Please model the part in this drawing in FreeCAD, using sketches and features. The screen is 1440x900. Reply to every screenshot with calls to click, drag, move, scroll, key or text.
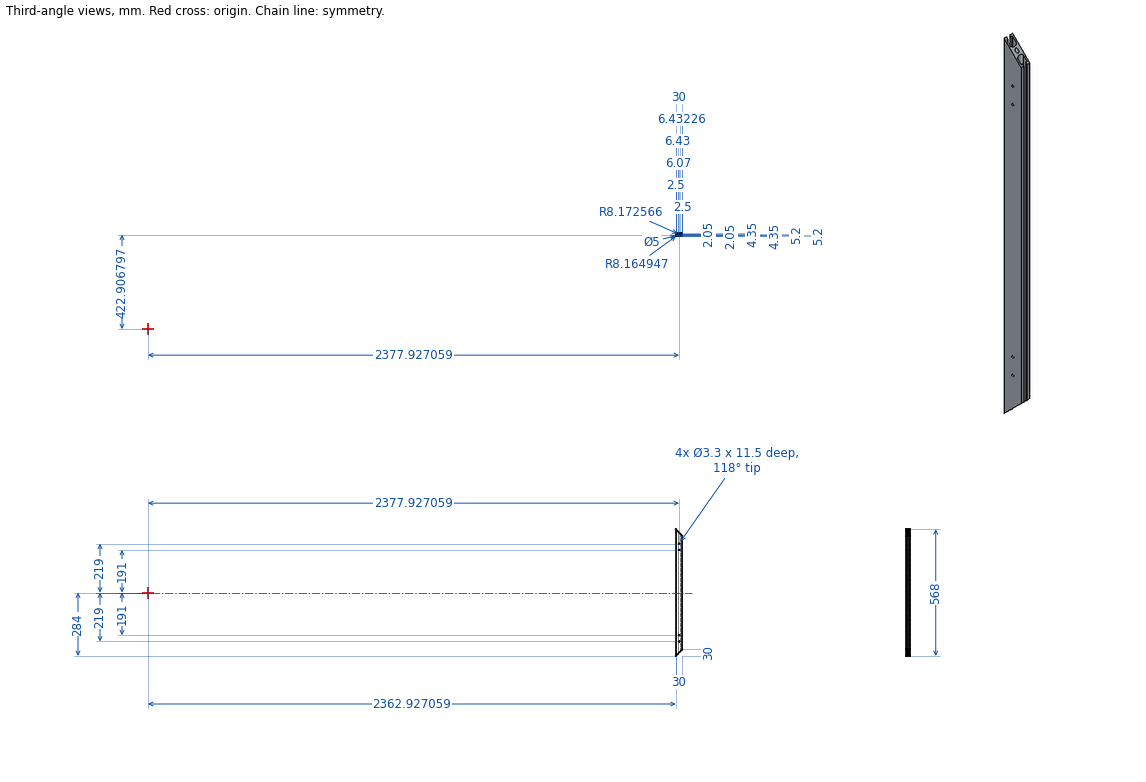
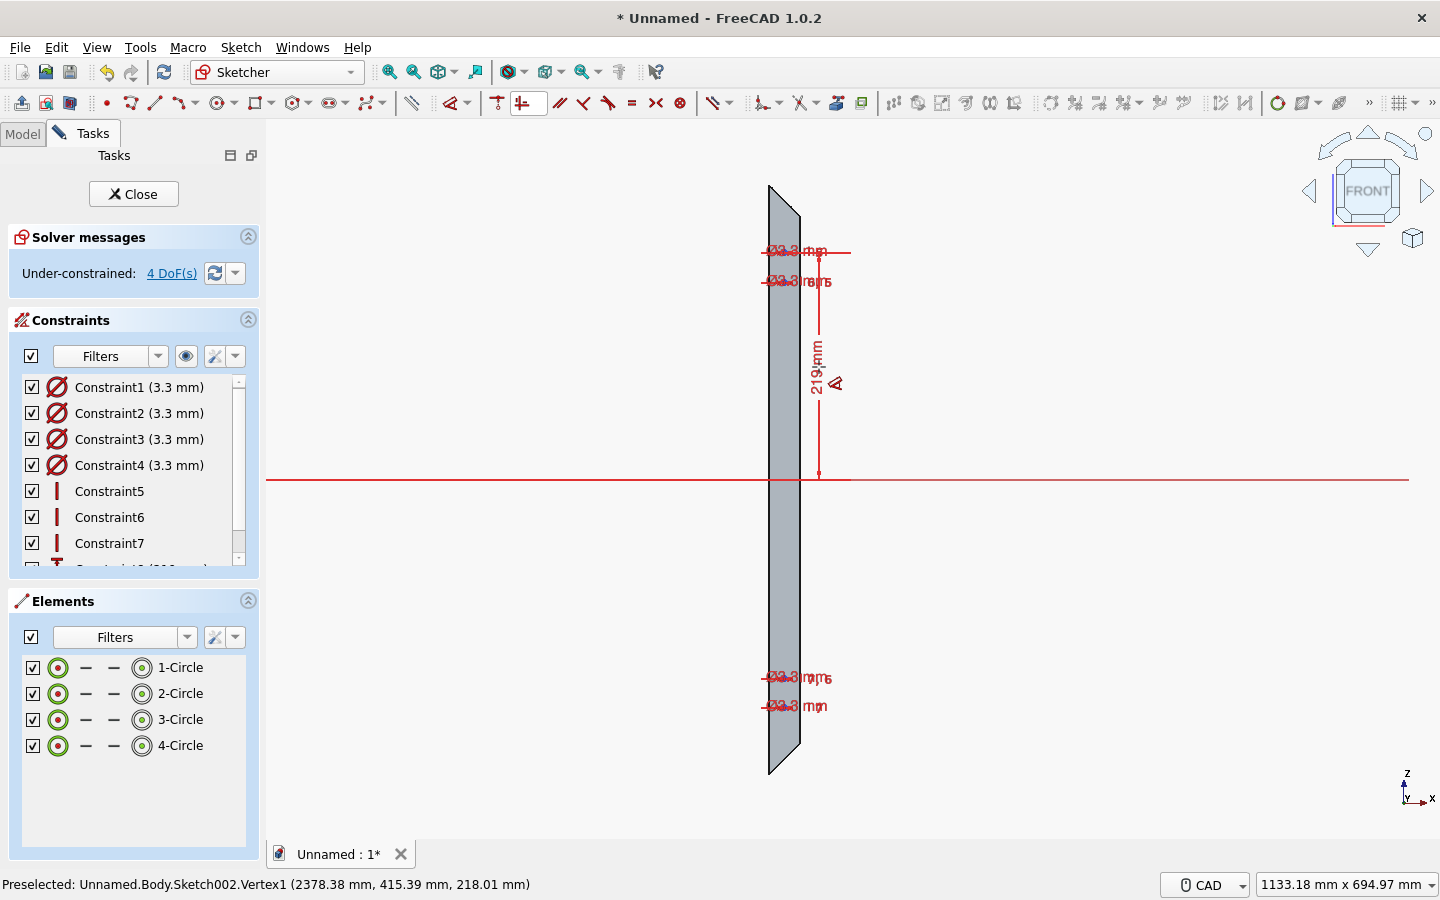
click(785, 283)
click(819, 336)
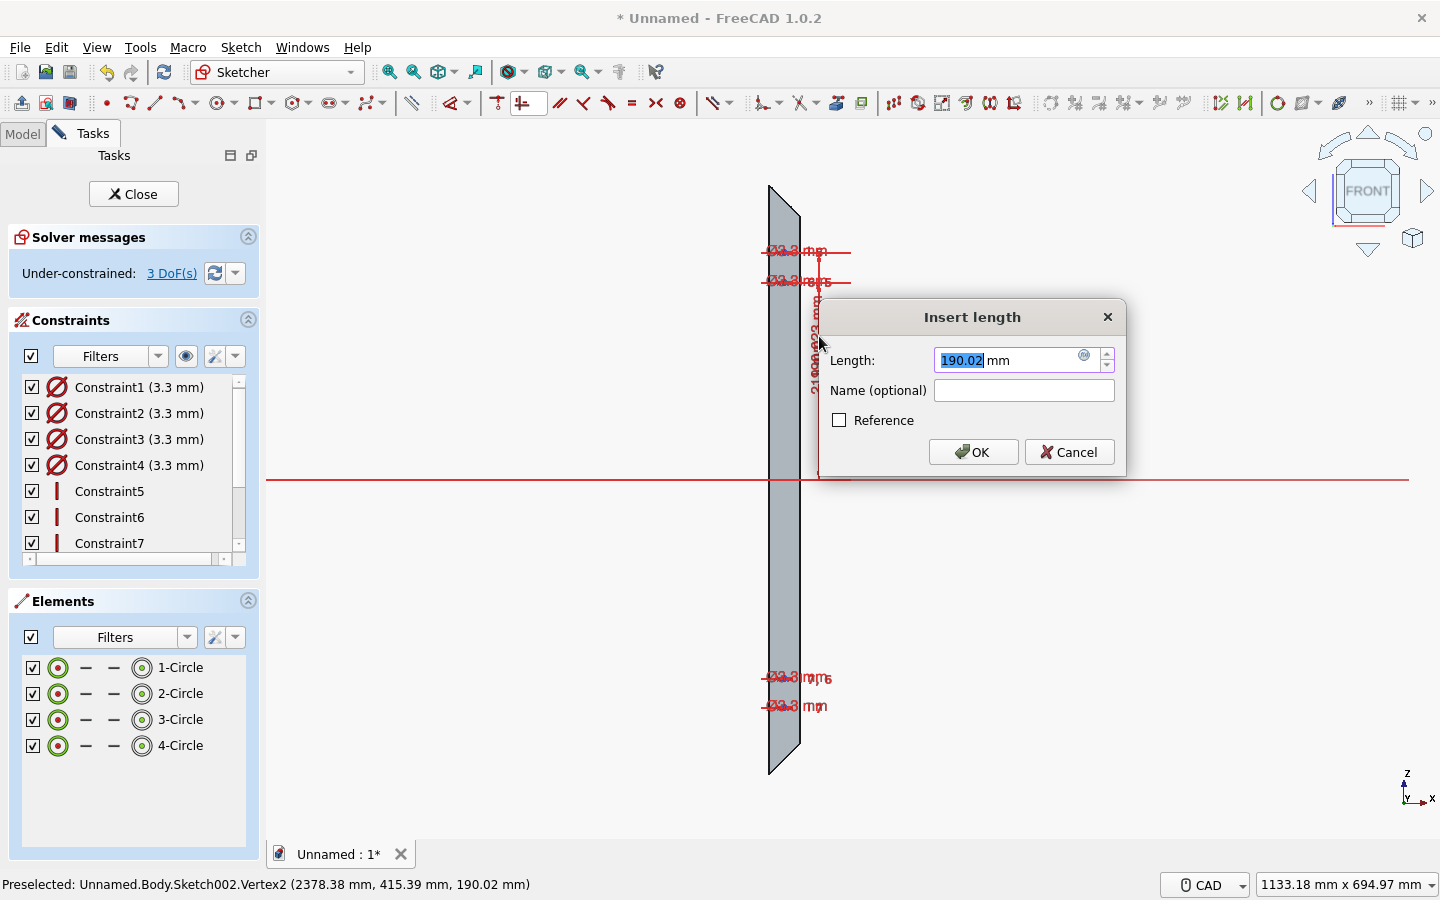
text(191)
key(Return)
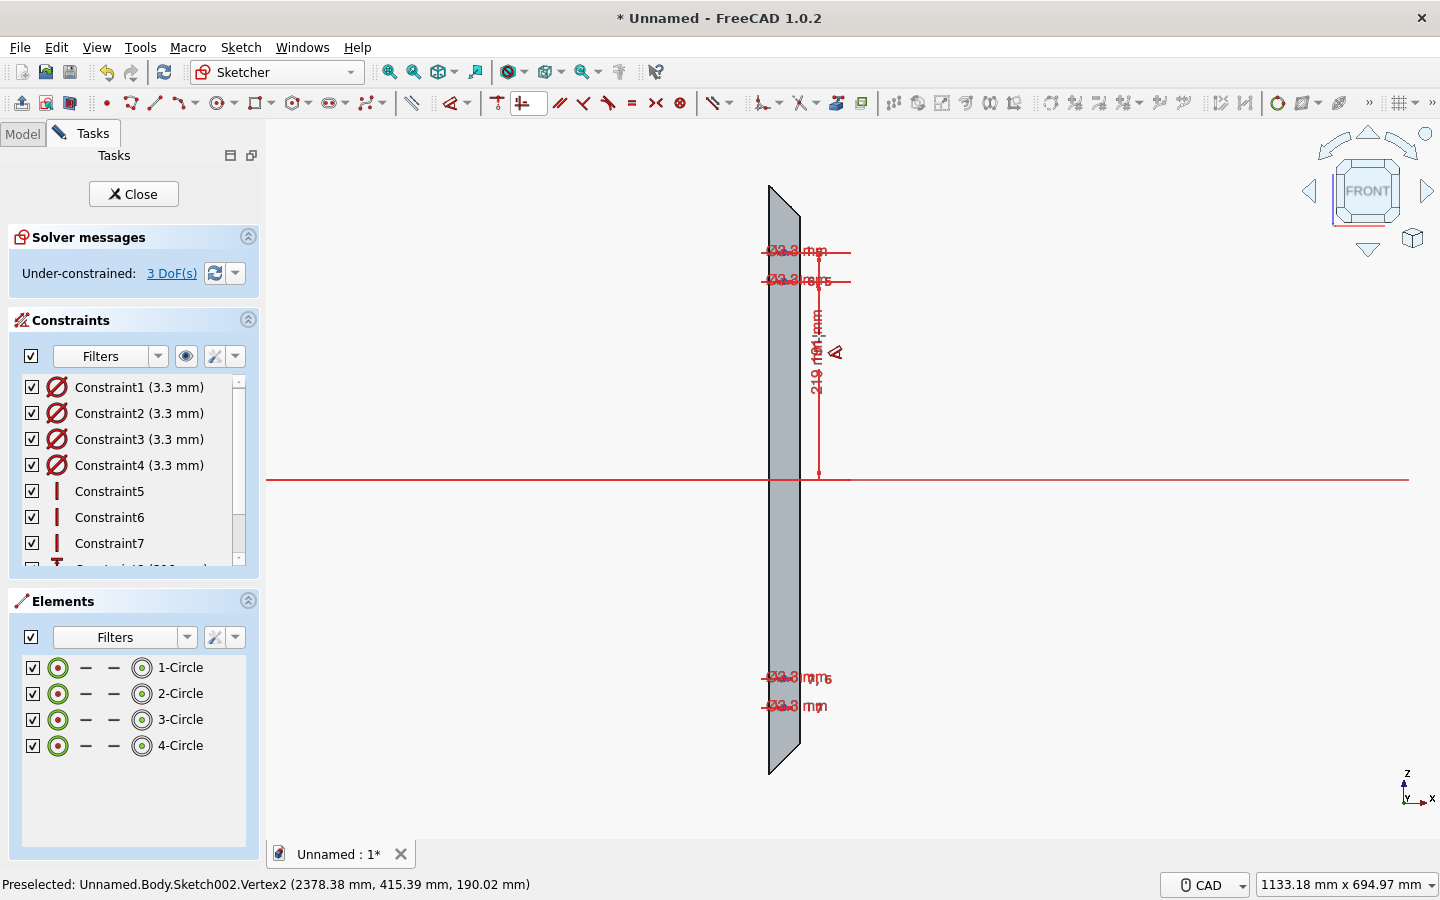
click(785, 679)
click(819, 579)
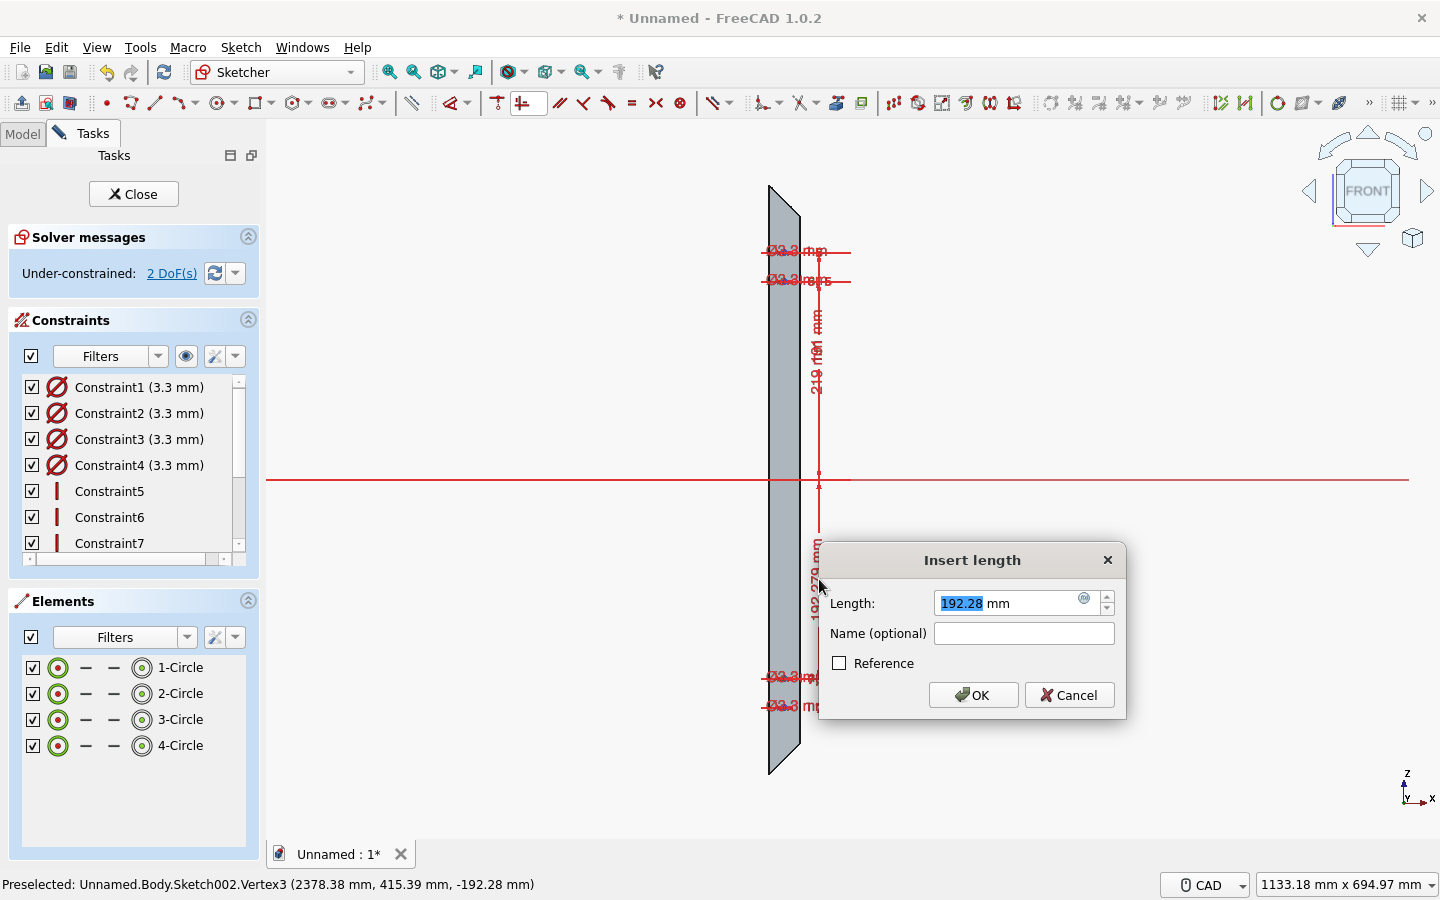
text(191)
key(Return)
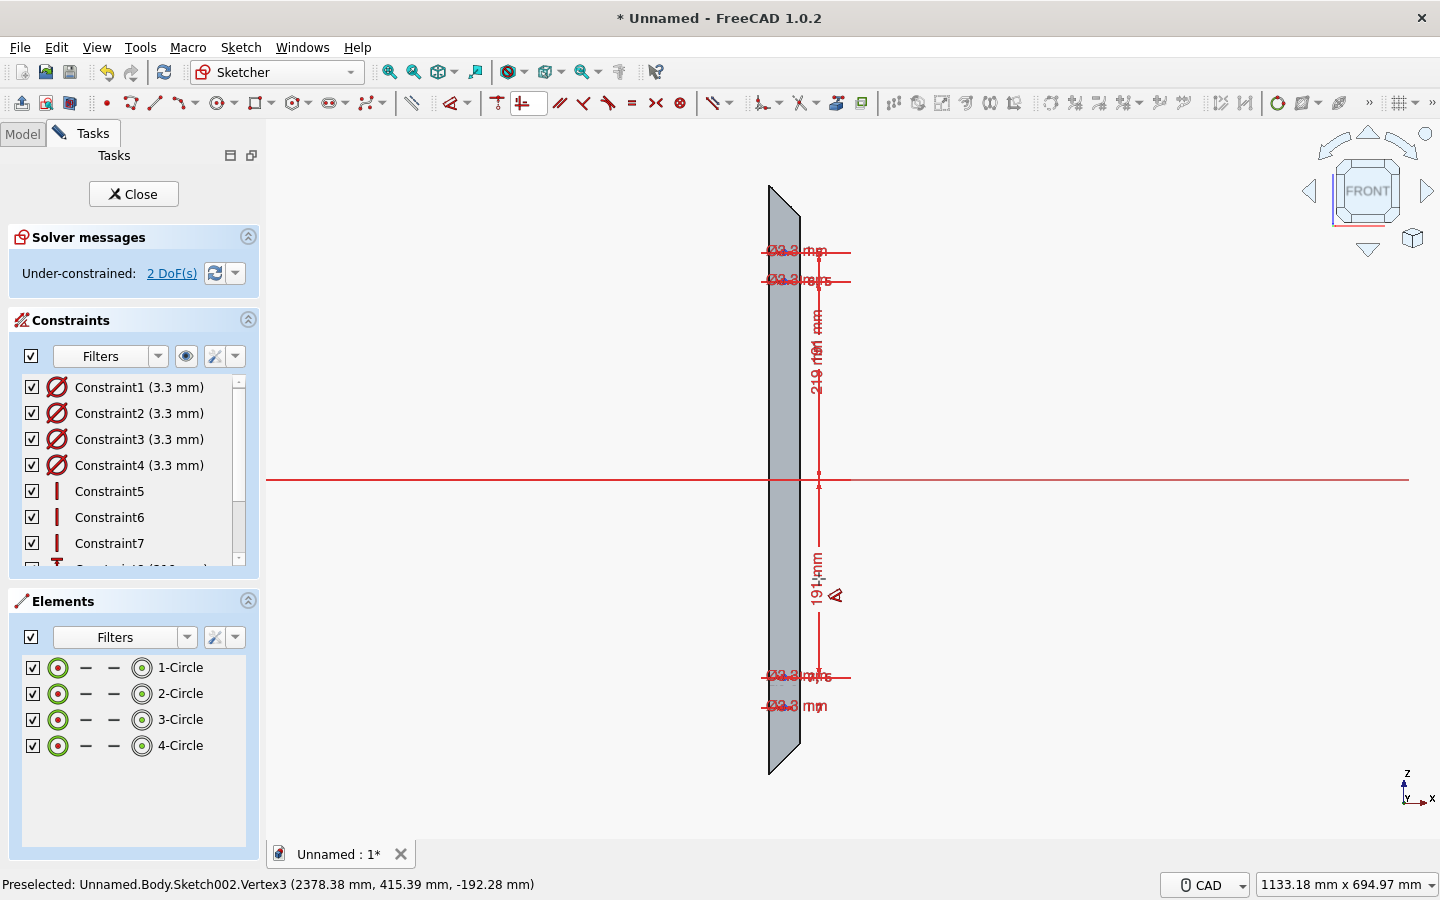
click(785, 708)
click(819, 541)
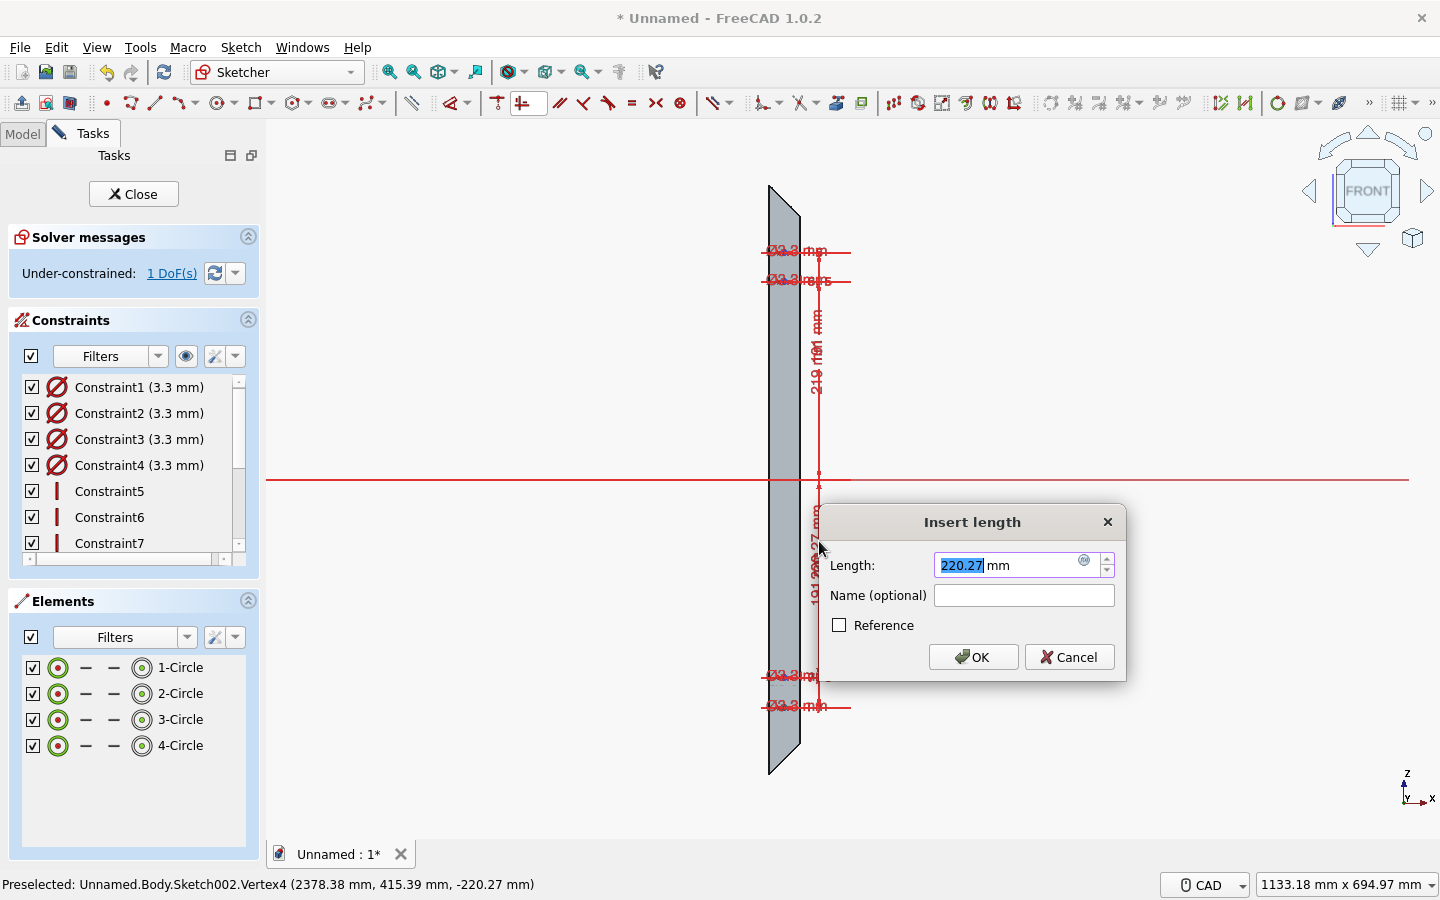
text(219)
key(Return)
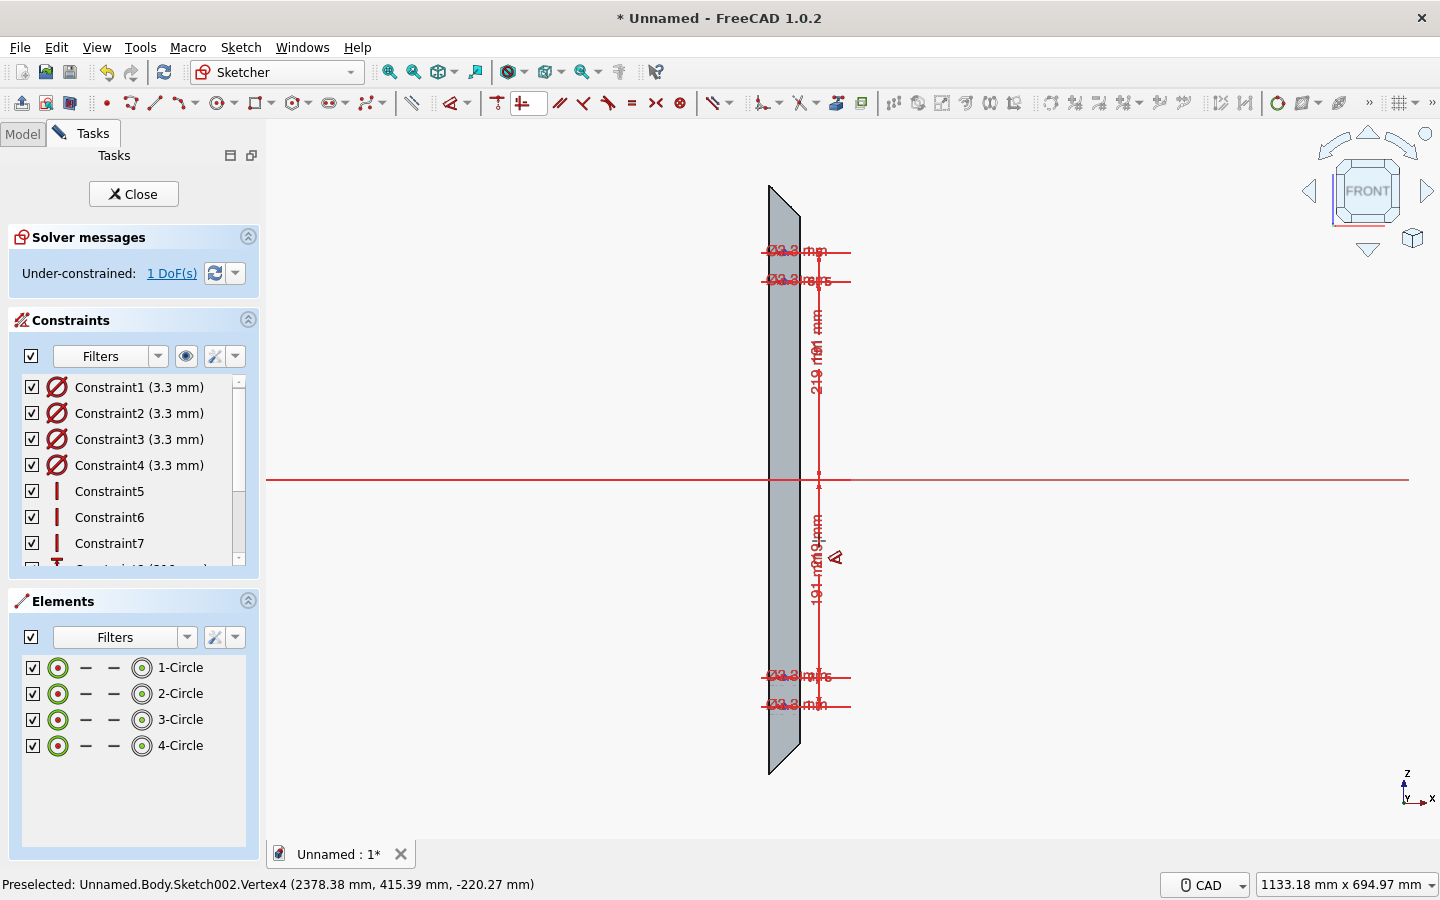
click(785, 253)
click(539, 219)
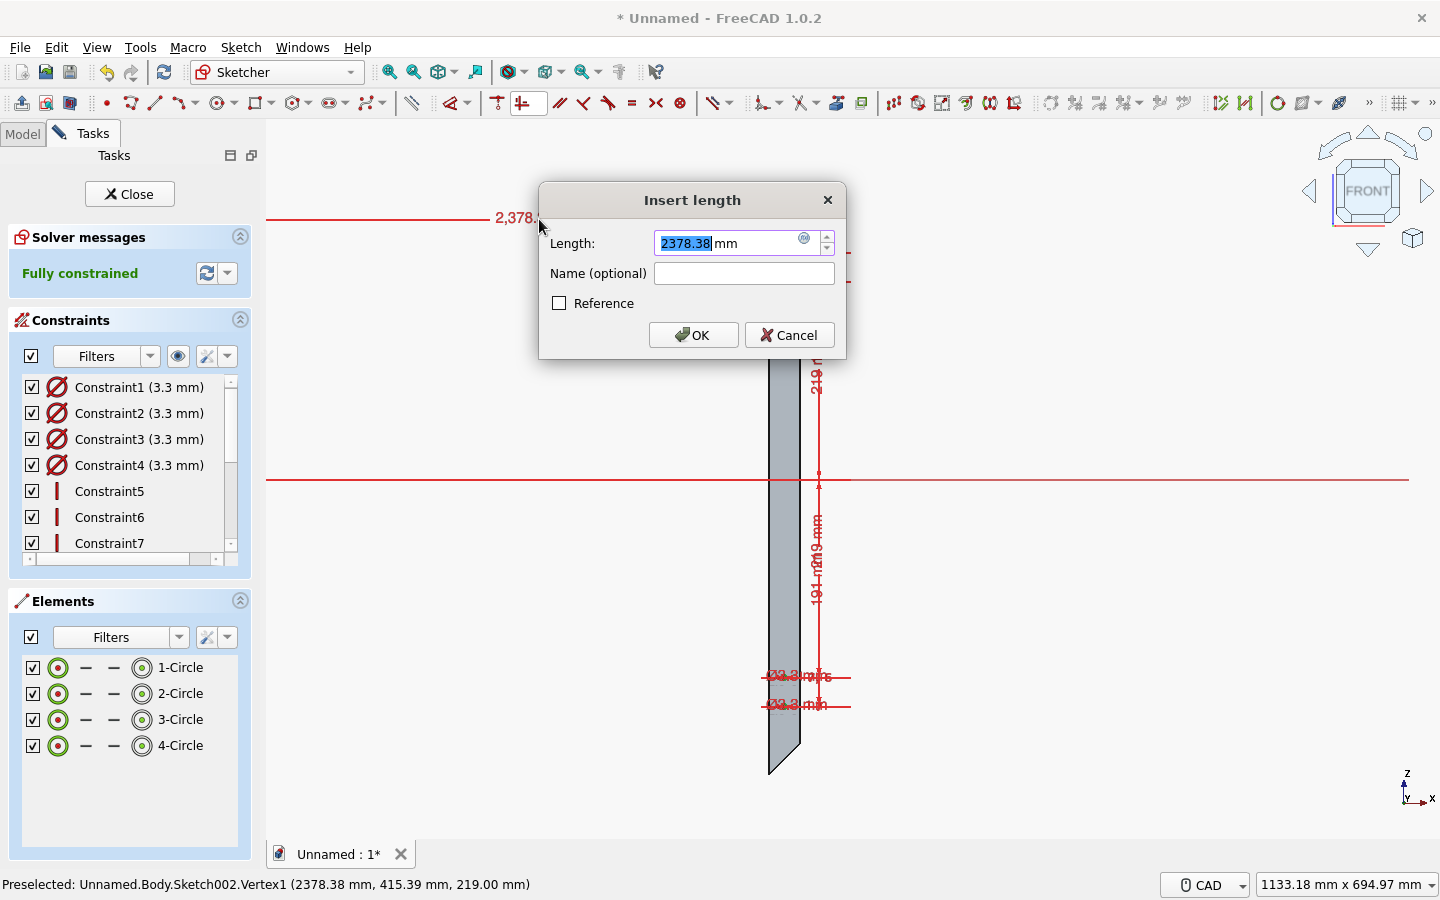
text(2377.927059)
key(Return)
key(Escape)